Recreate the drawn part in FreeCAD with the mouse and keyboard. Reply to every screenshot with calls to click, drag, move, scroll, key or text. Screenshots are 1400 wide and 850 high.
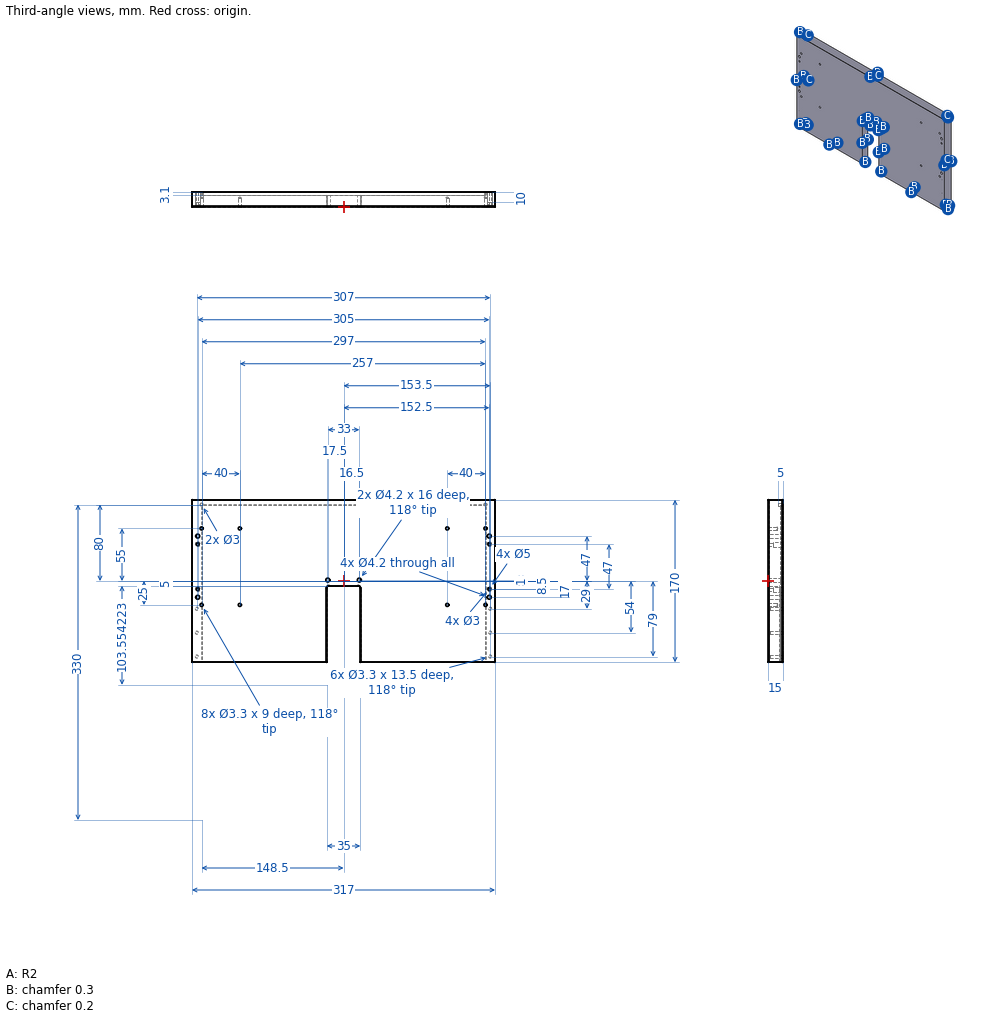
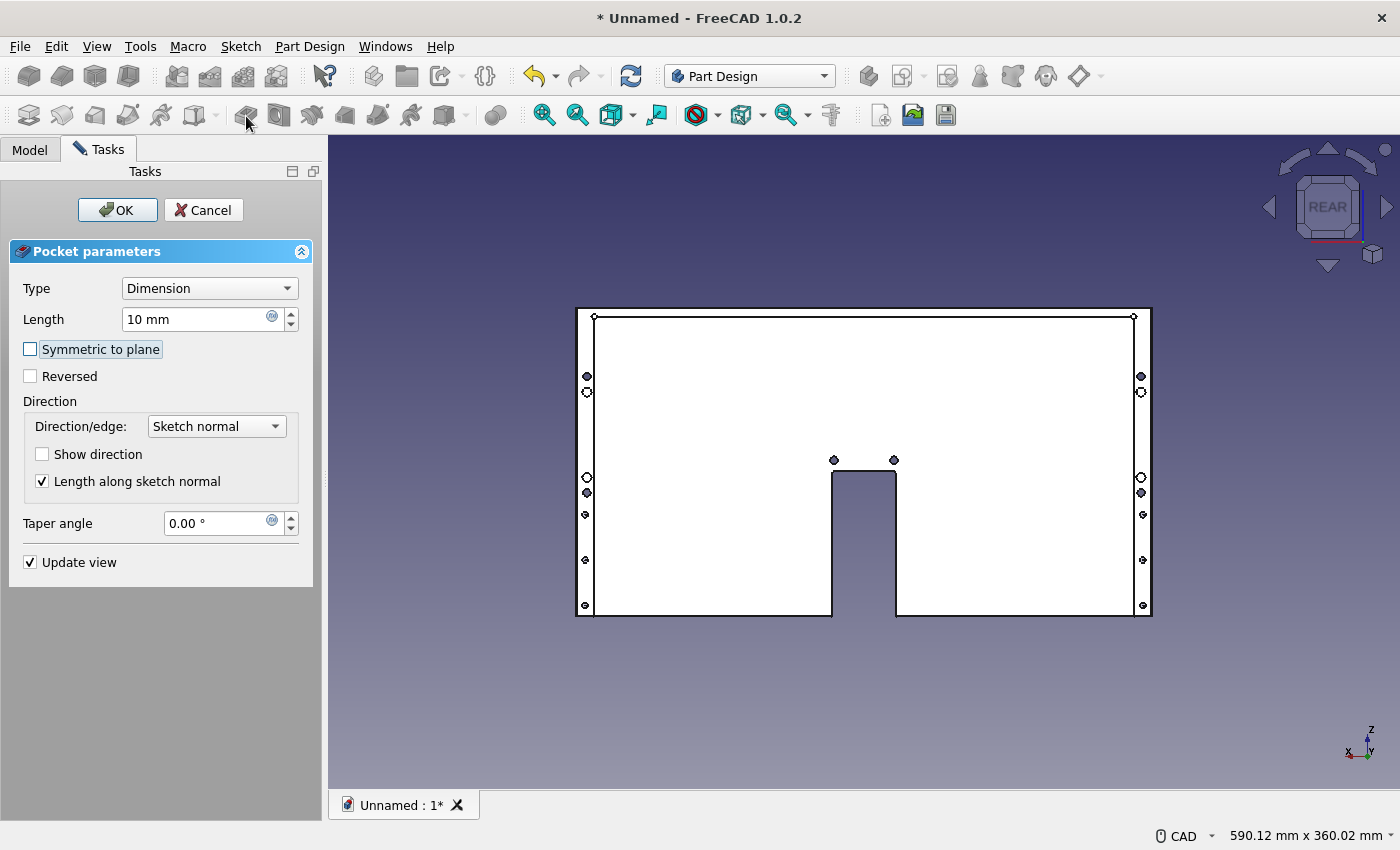
click(118, 210)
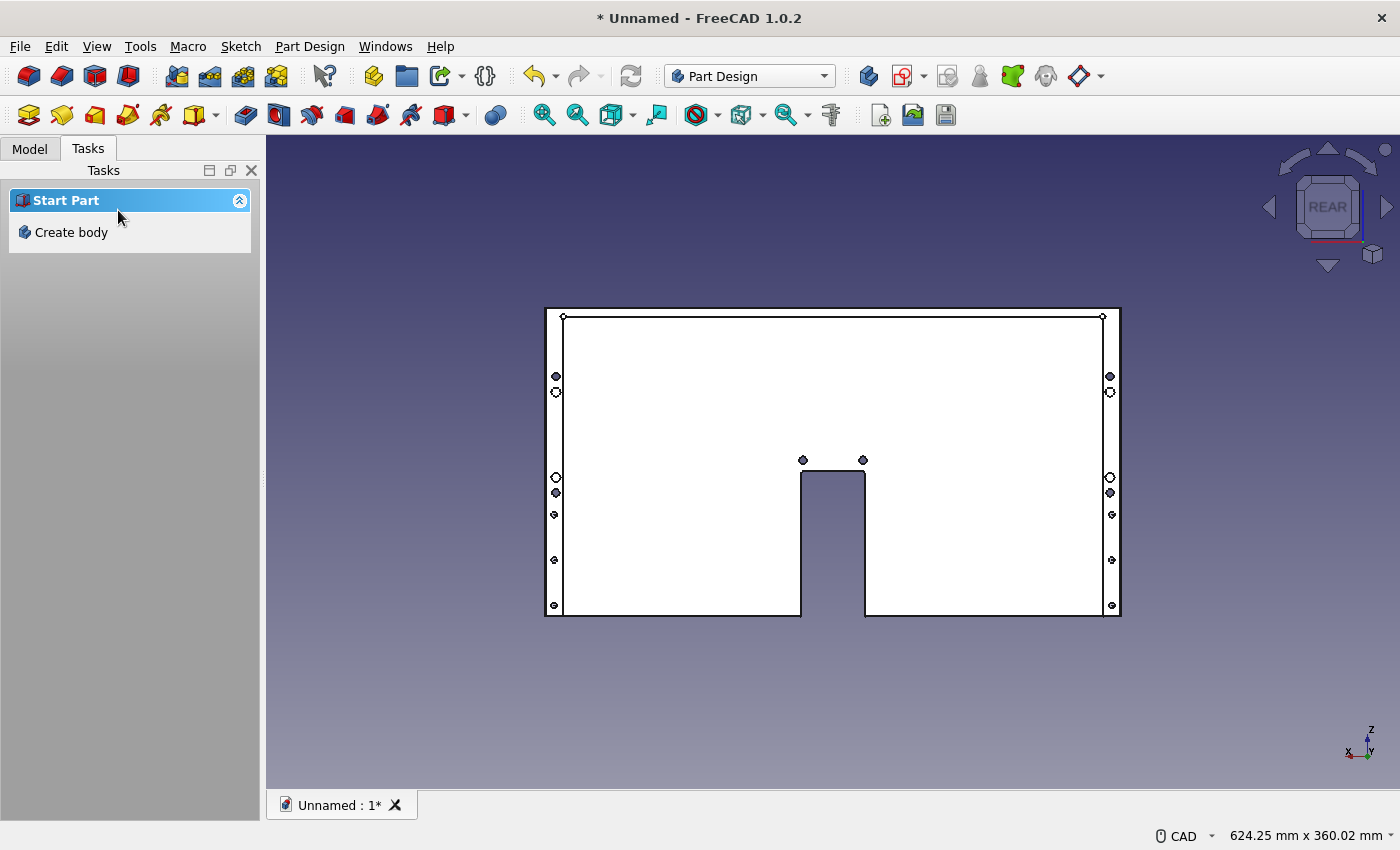
click(554, 575)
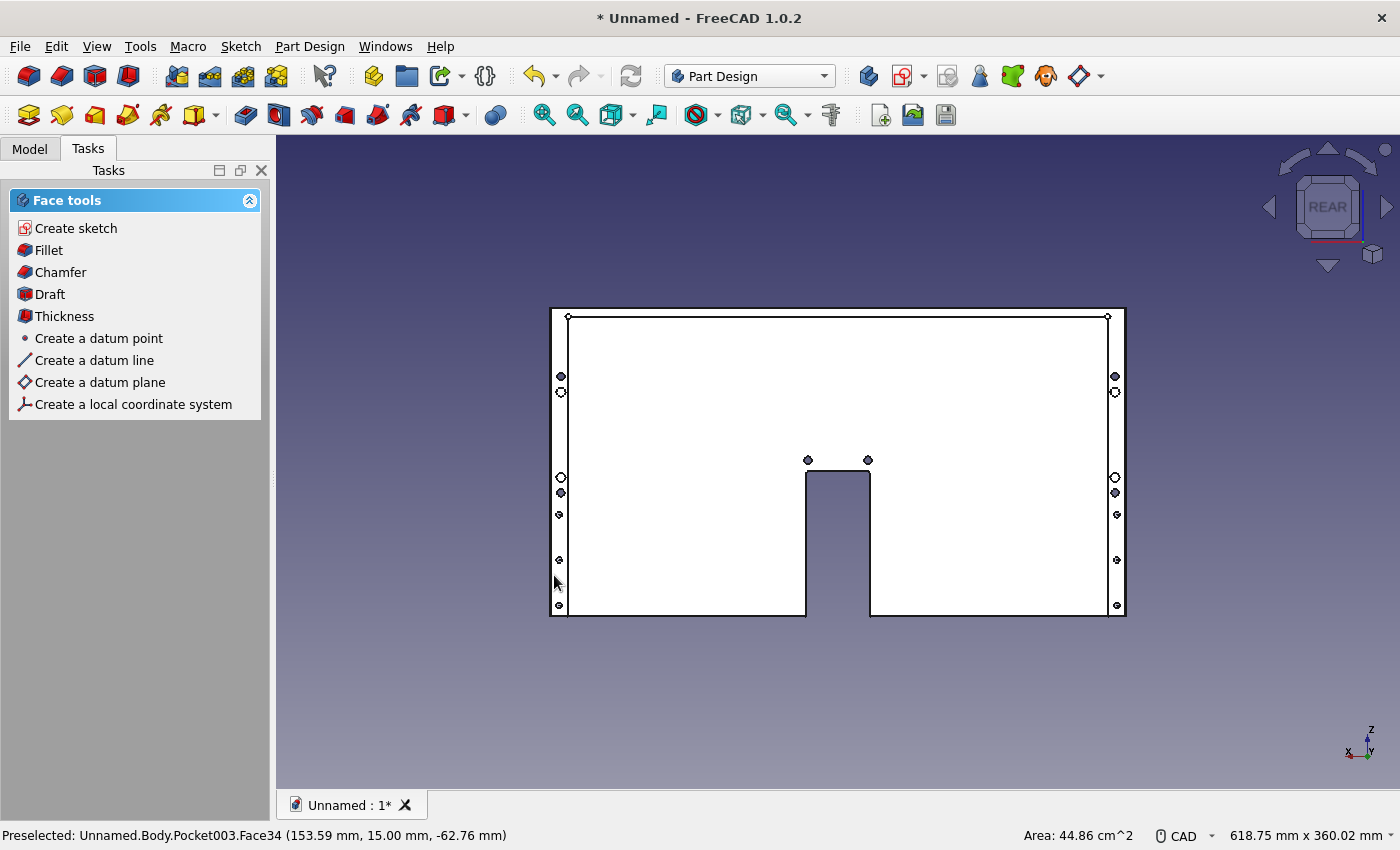
click(902, 76)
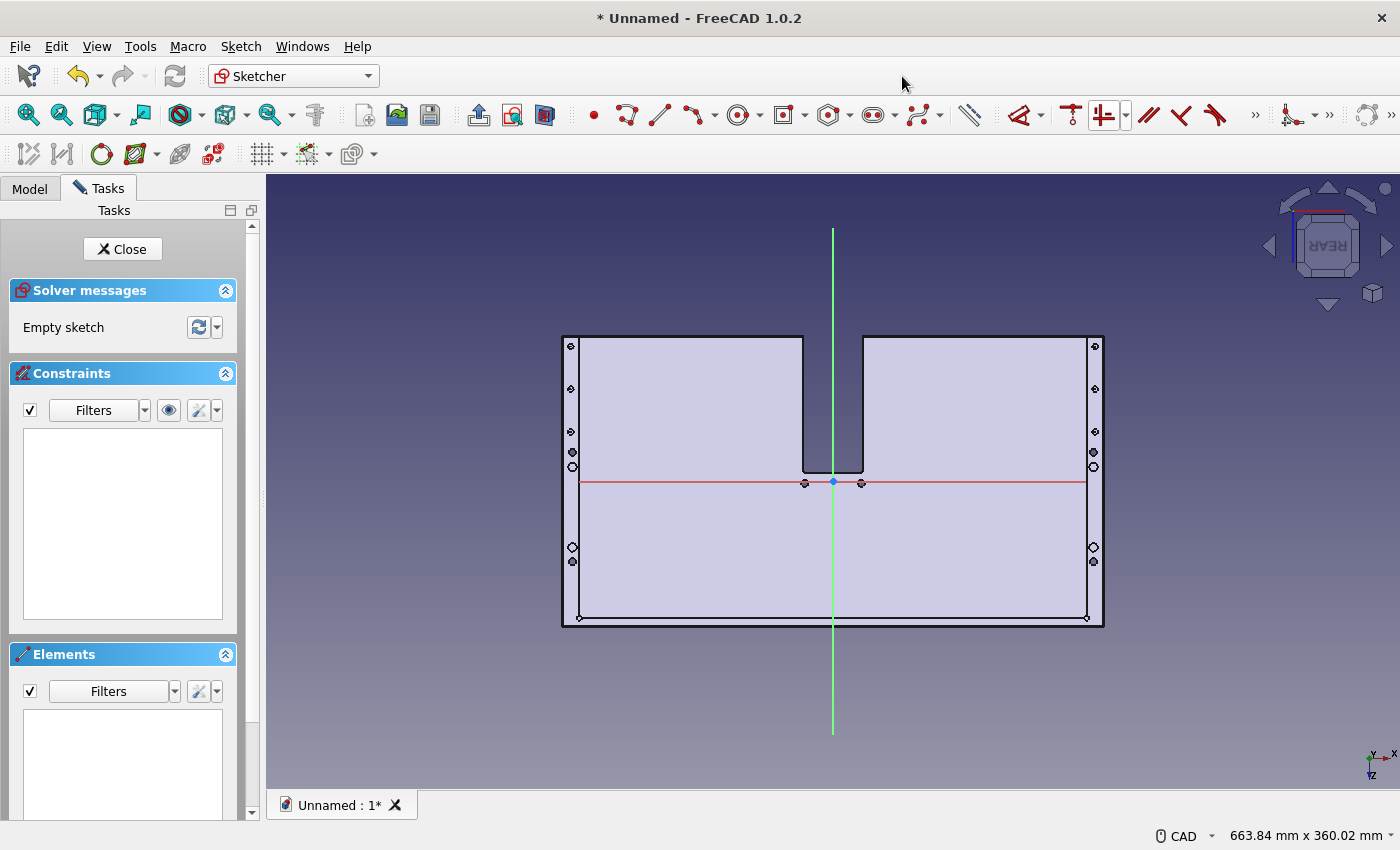
key(g)
key(c)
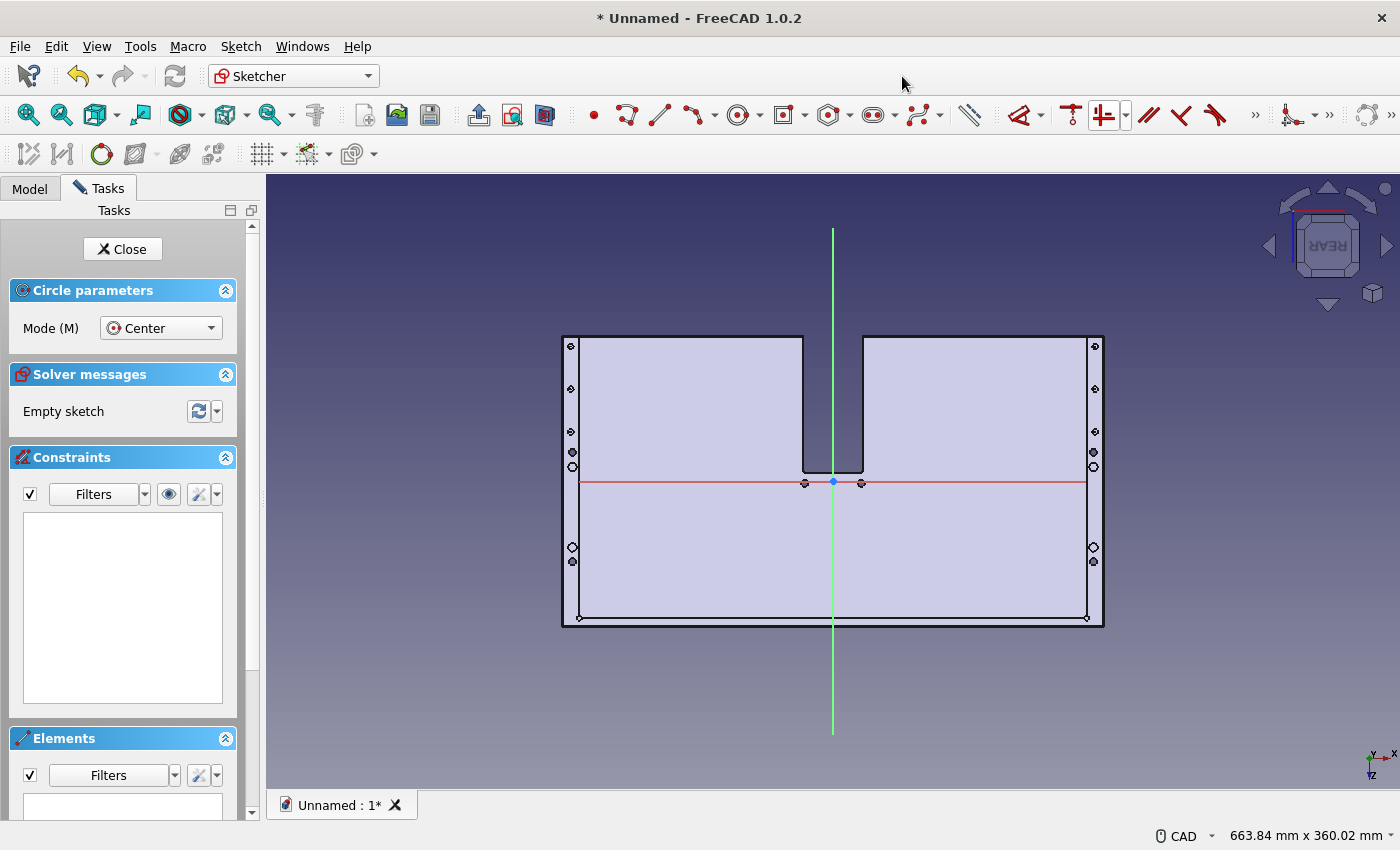
scroll(1094, 467, up, 11)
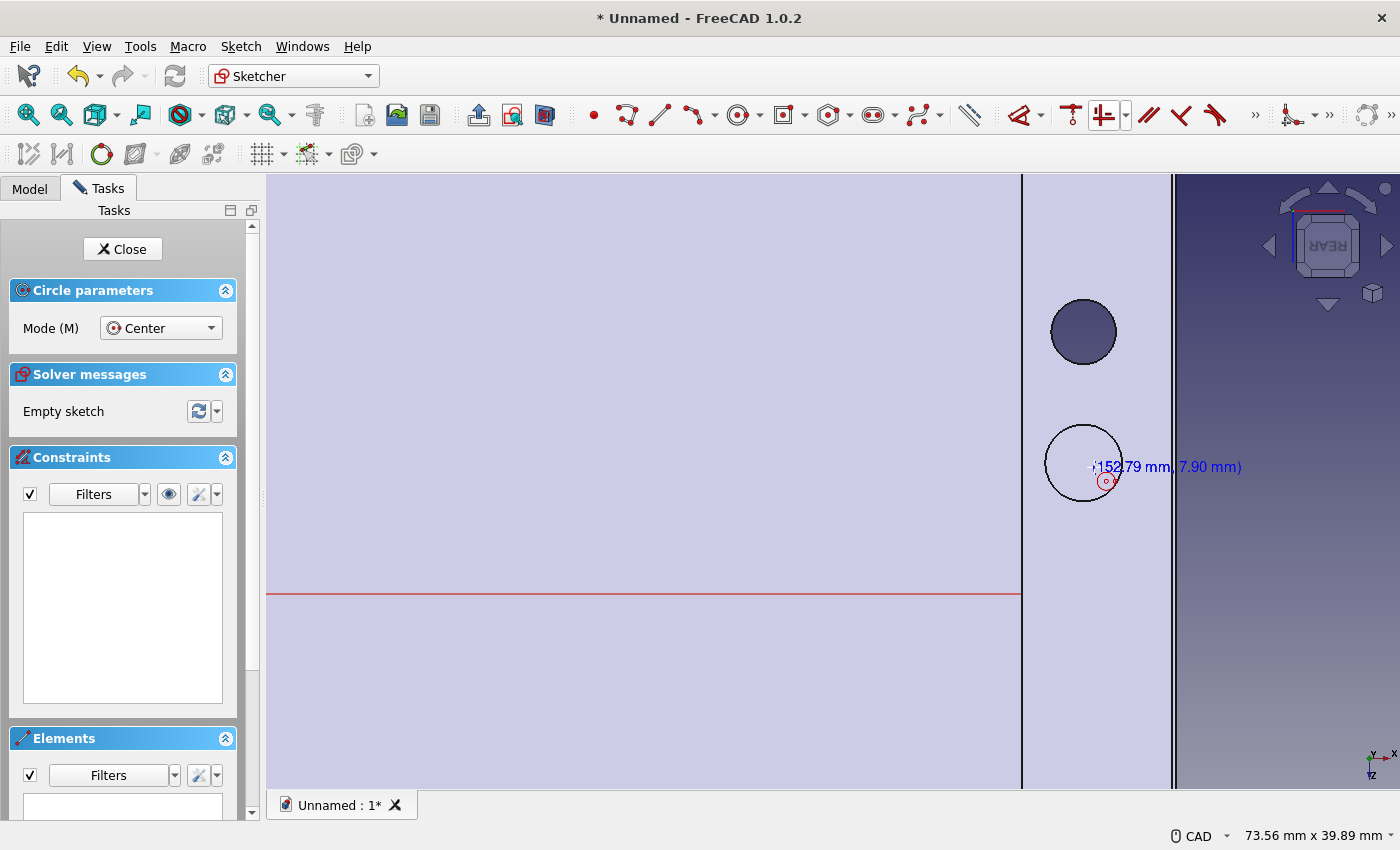
scroll(1083, 428, down, 10)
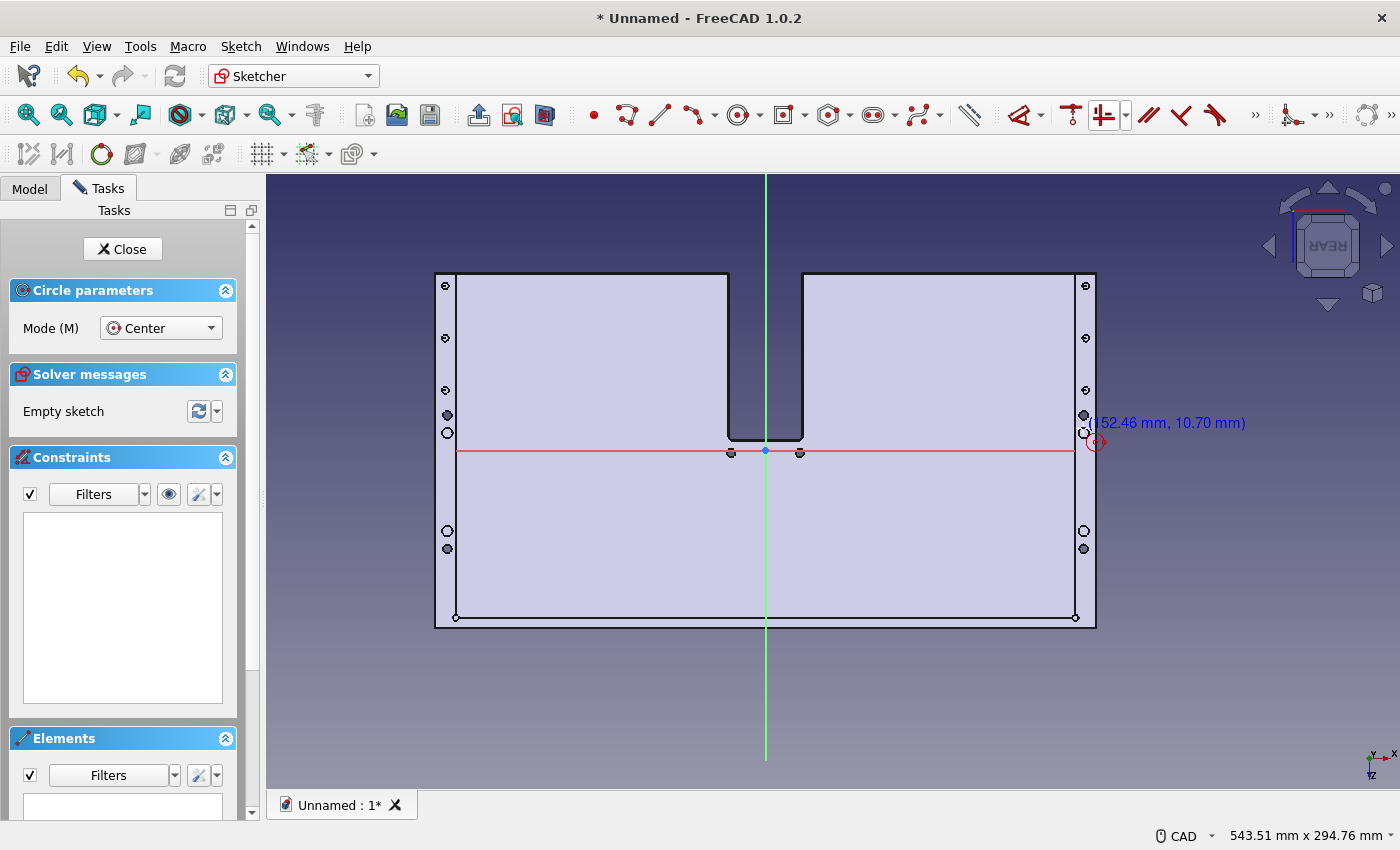
click(1084, 433)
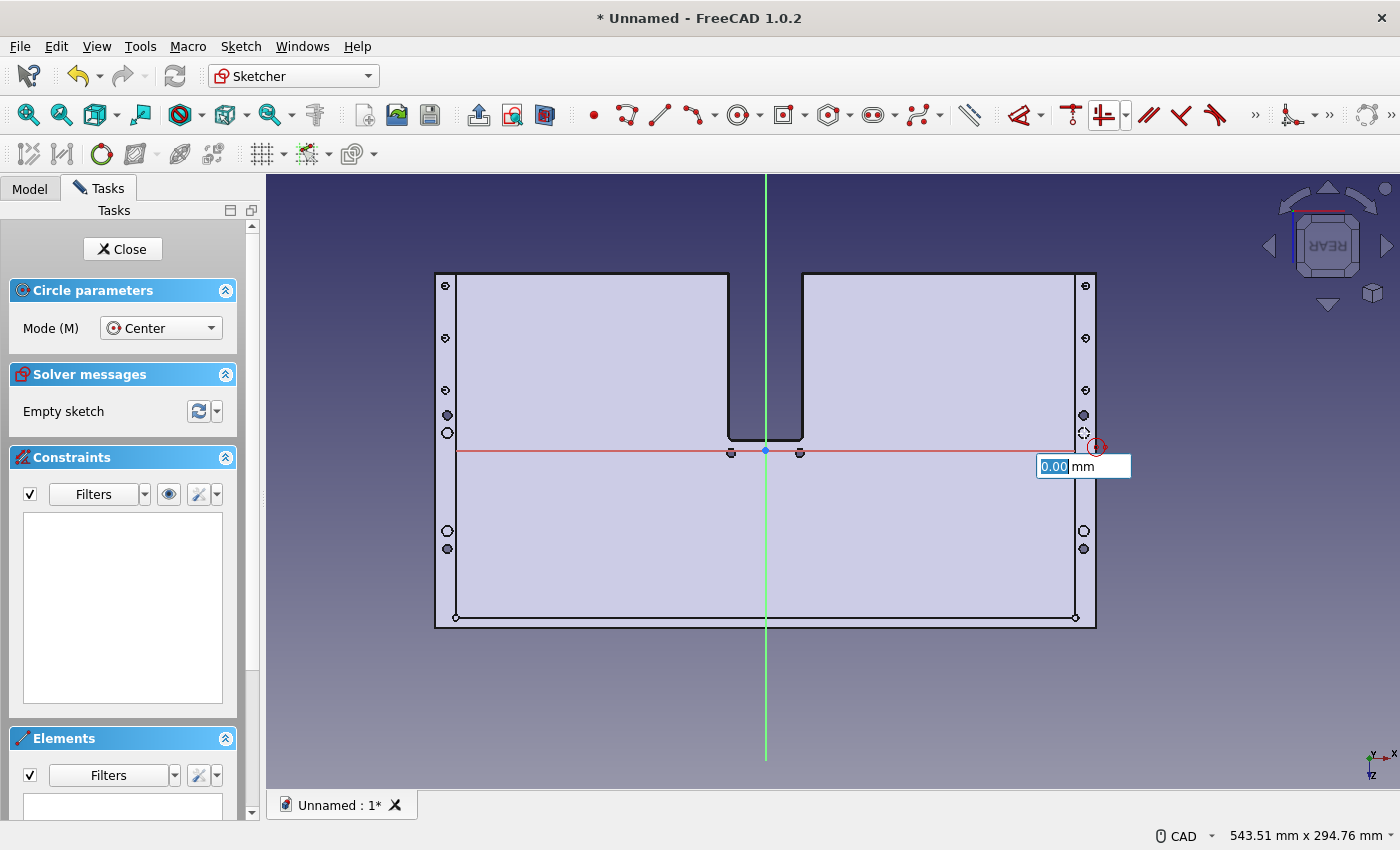
scroll(1086, 431, up, 9)